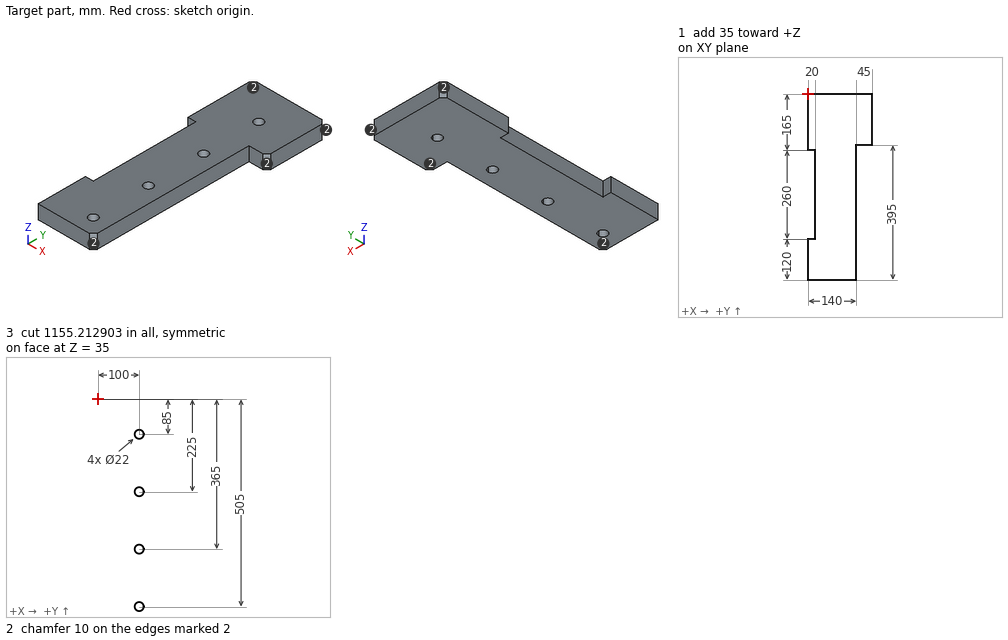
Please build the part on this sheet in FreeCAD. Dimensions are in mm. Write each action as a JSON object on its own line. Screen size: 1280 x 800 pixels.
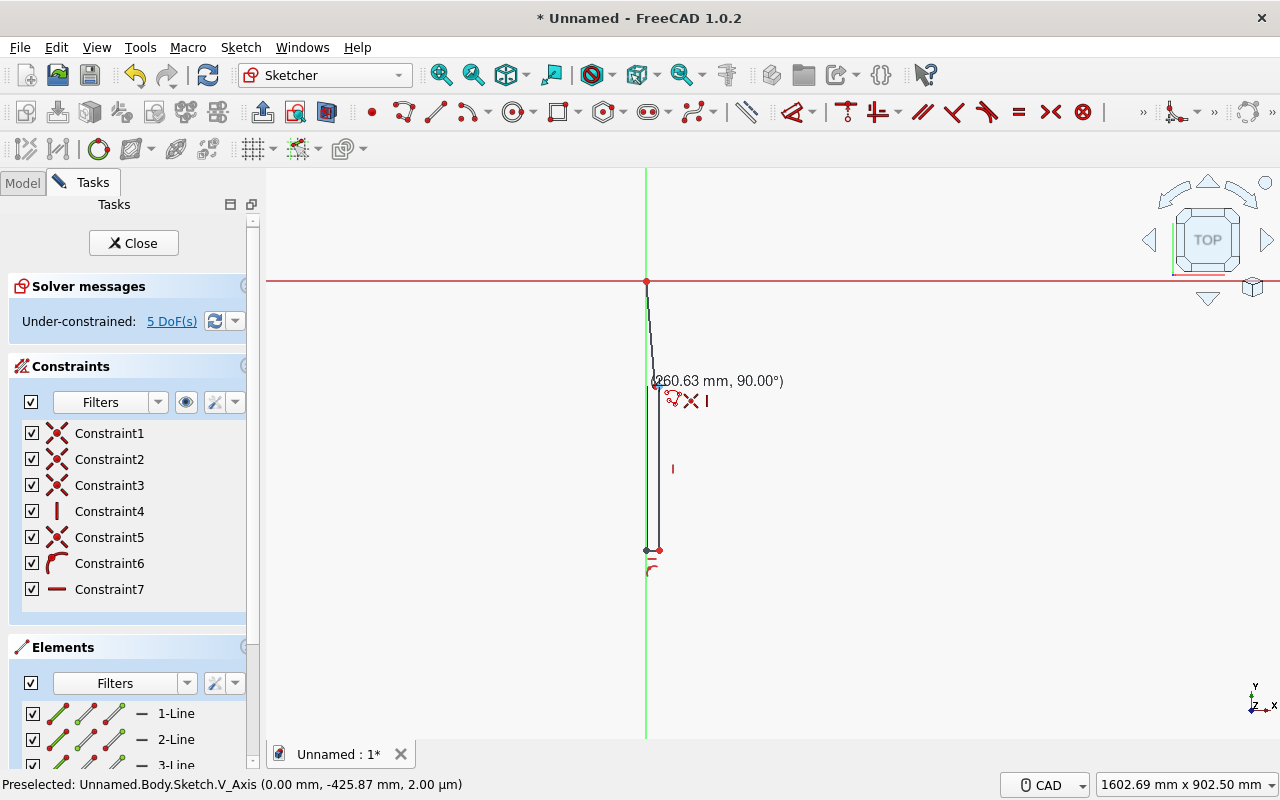
{"action": "left_click", "coordinate": [655, 626]}
{"action": "left_click", "coordinate": [735, 626]}
{"action": "left_click", "coordinate": [735, 376]}
{"action": "left_click", "coordinate": [763, 376]}
{"action": "left_click", "coordinate": [763, 290]}
{"action": "left_click", "coordinate": [646, 281]}
{"action": "key", "text": "Escape"}
{"action": "key", "text": "Escape"}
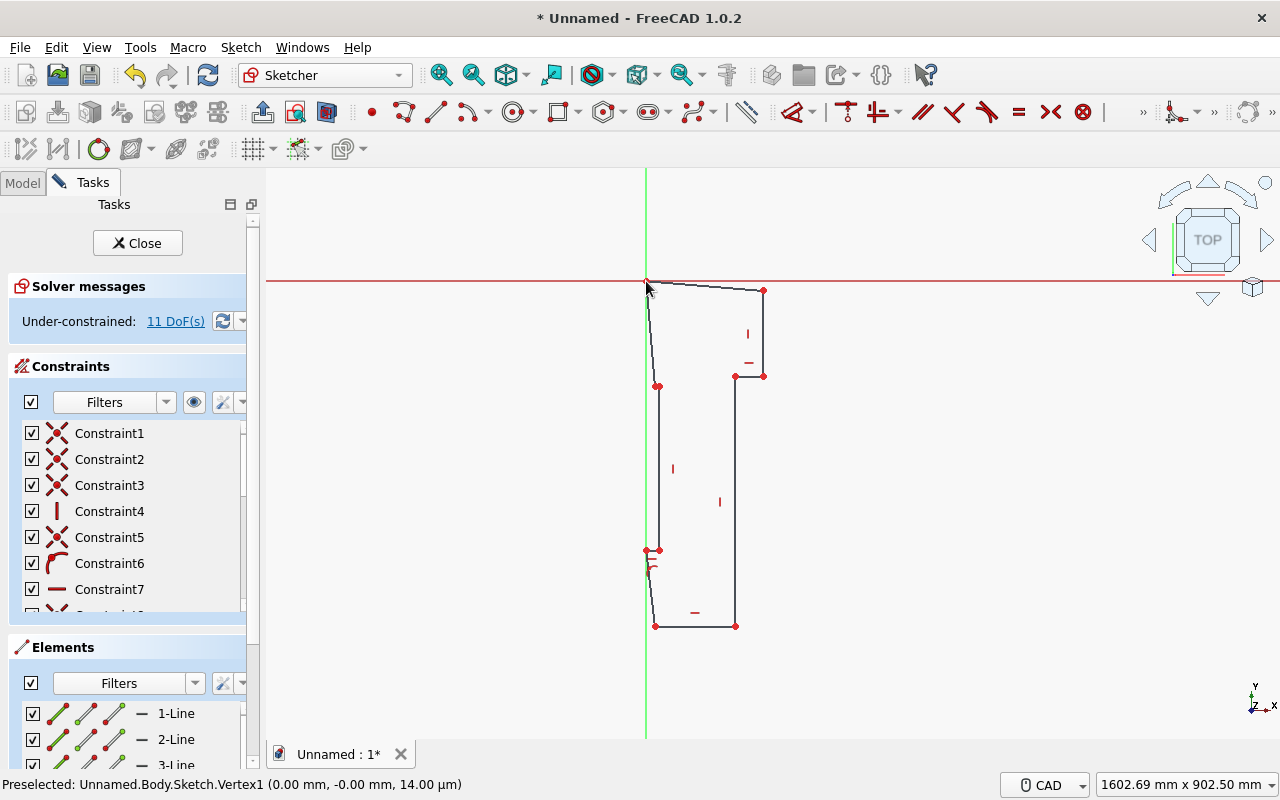
{"action": "left_click", "coordinate": [649, 313]}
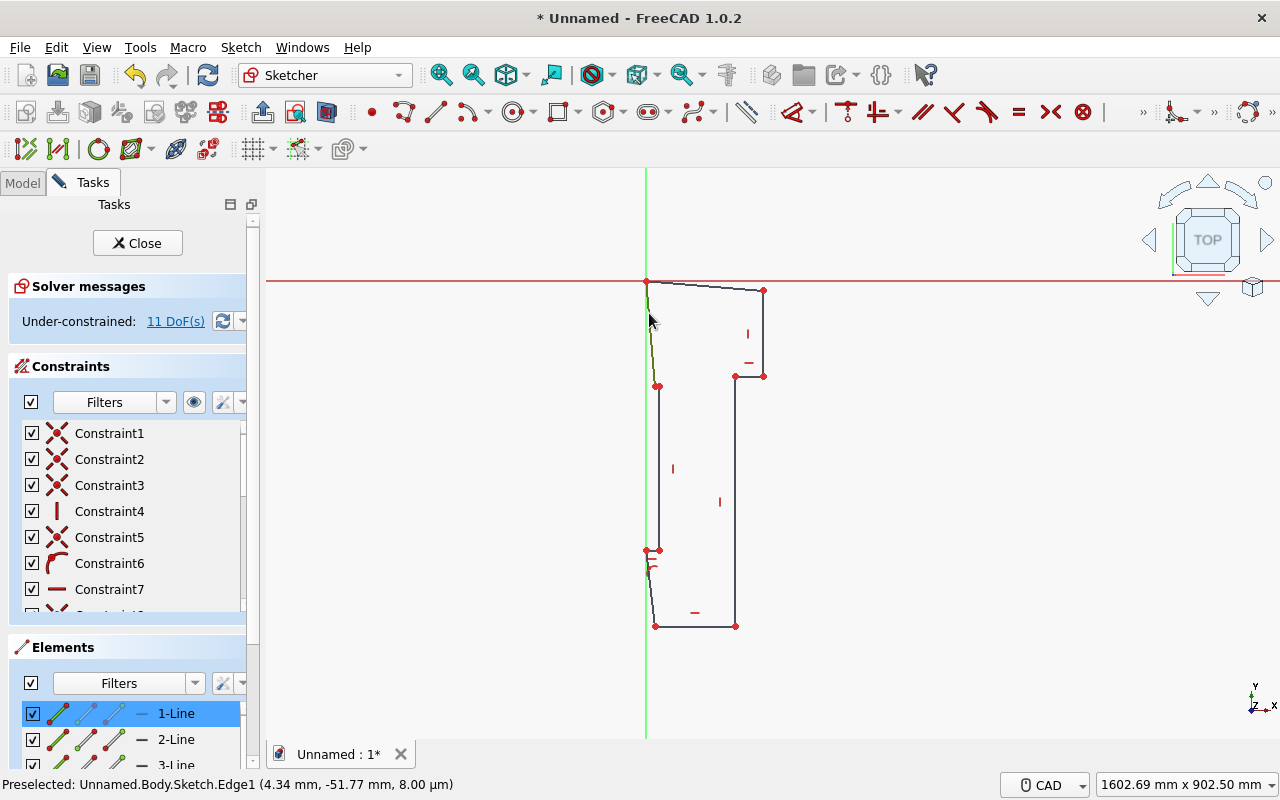
{"action": "left_click", "coordinate": [900, 112]}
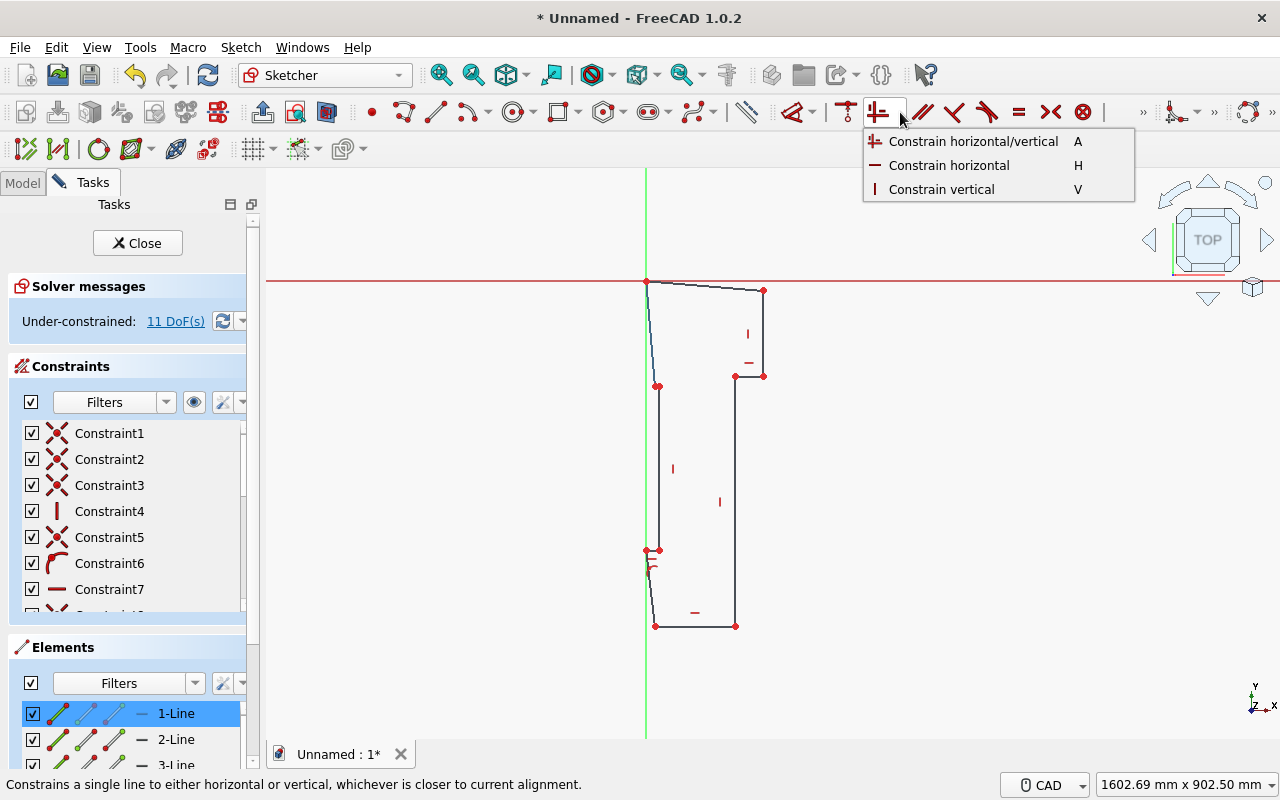
{"action": "left_click", "coordinate": [999, 189]}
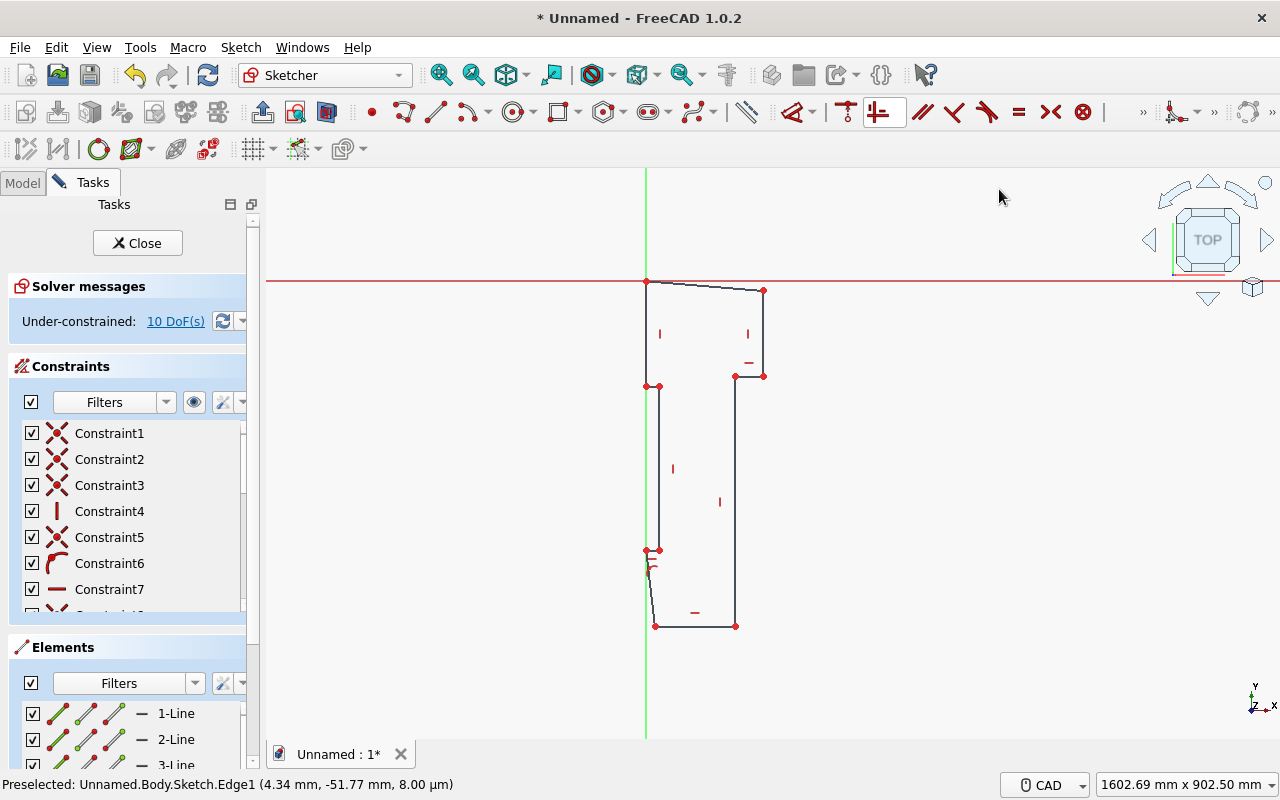
{"action": "scroll", "coordinate": [653, 387], "scroll_direction": "up", "scroll_amount": 4}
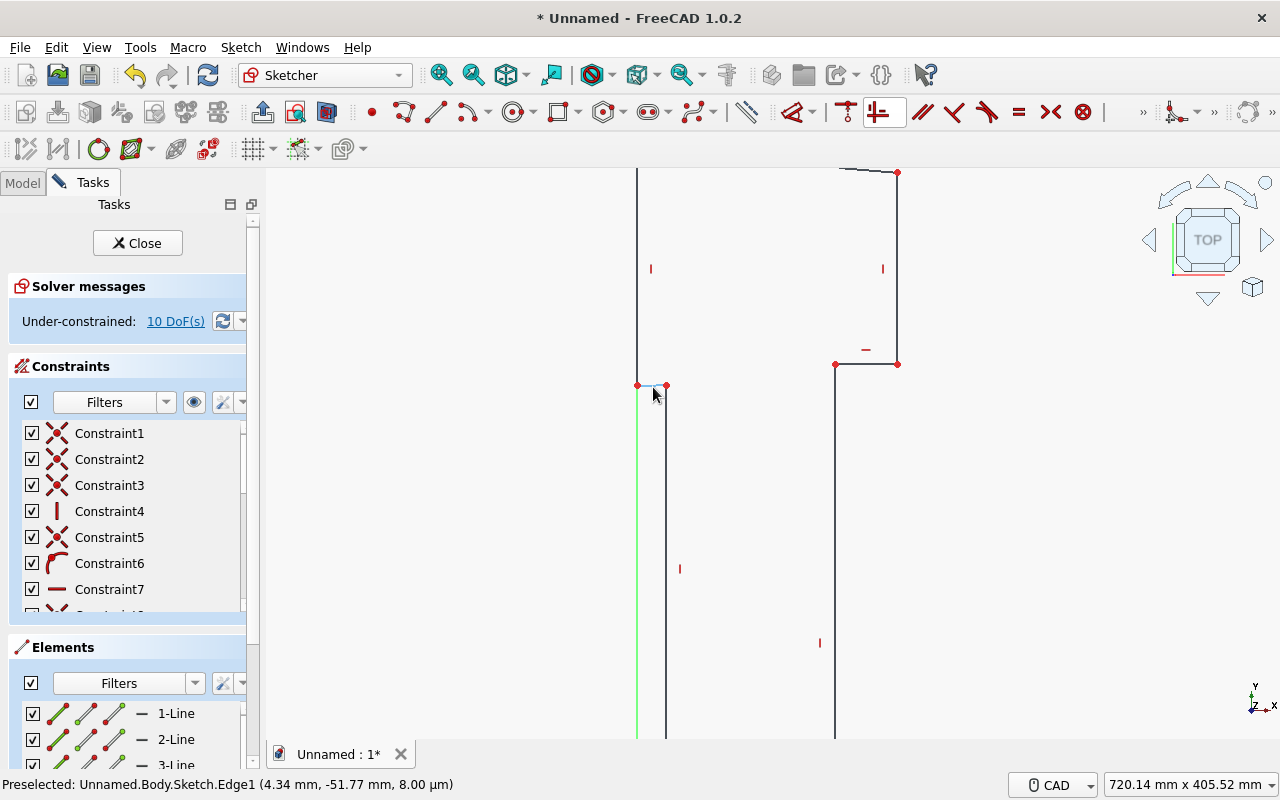
{"action": "left_click", "coordinate": [652, 386]}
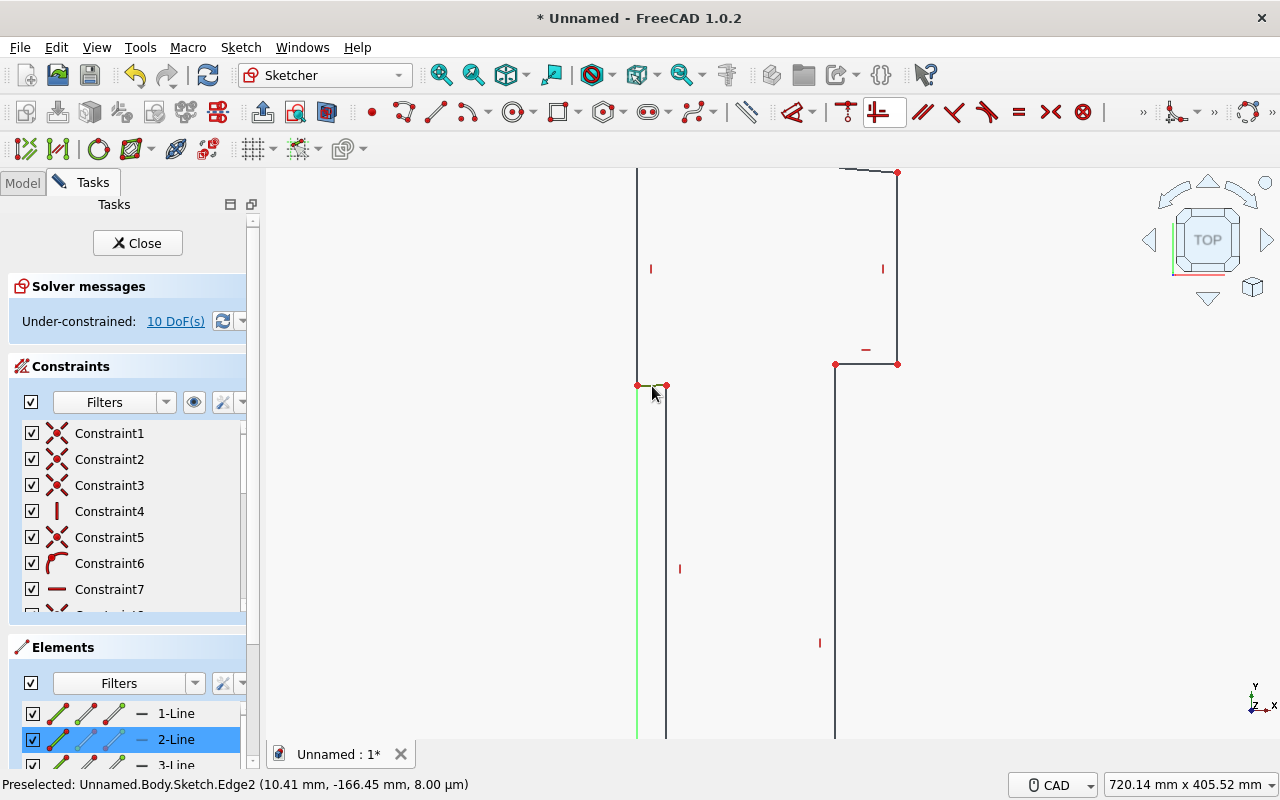
{"action": "key", "text": "h"}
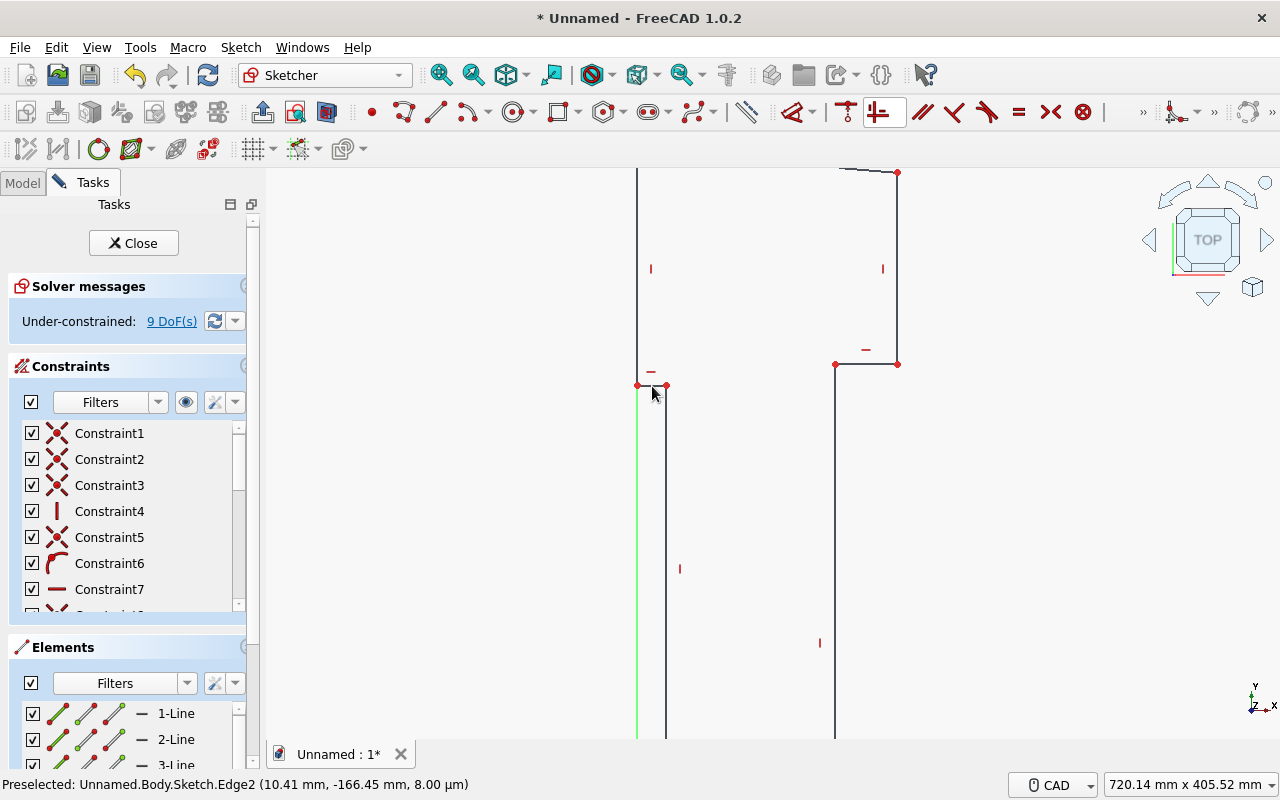
{"action": "scroll", "coordinate": [653, 387], "scroll_direction": "down", "scroll_amount": 4}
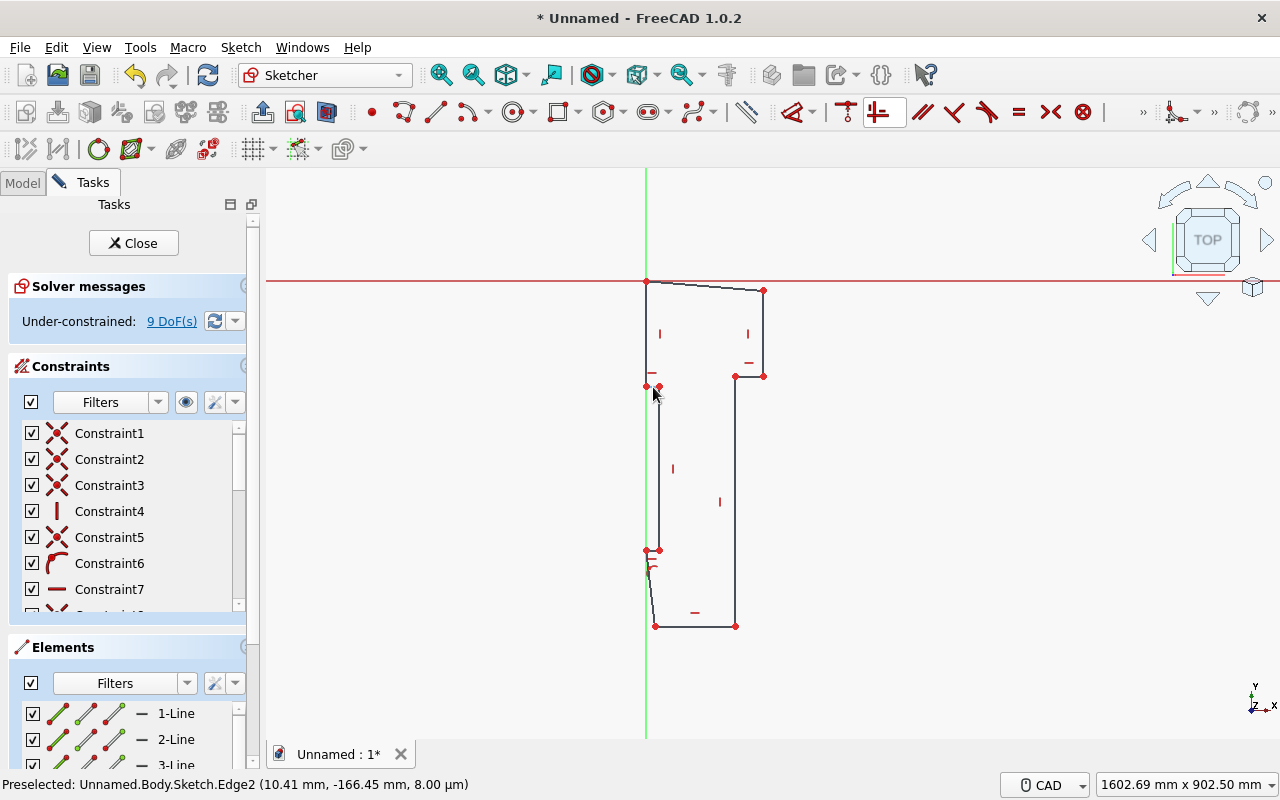
{"action": "scroll", "coordinate": [652, 604], "scroll_direction": "up", "scroll_amount": 5}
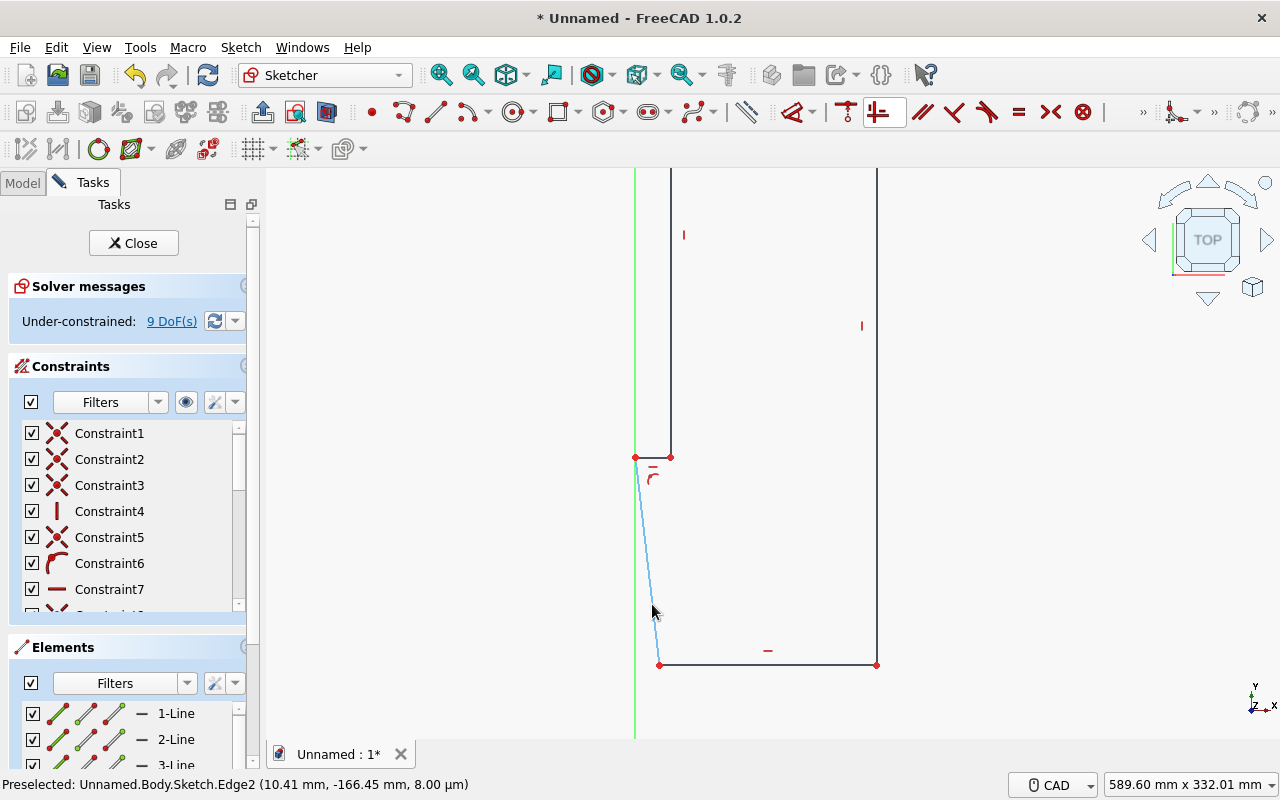
{"action": "left_click", "coordinate": [652, 603]}